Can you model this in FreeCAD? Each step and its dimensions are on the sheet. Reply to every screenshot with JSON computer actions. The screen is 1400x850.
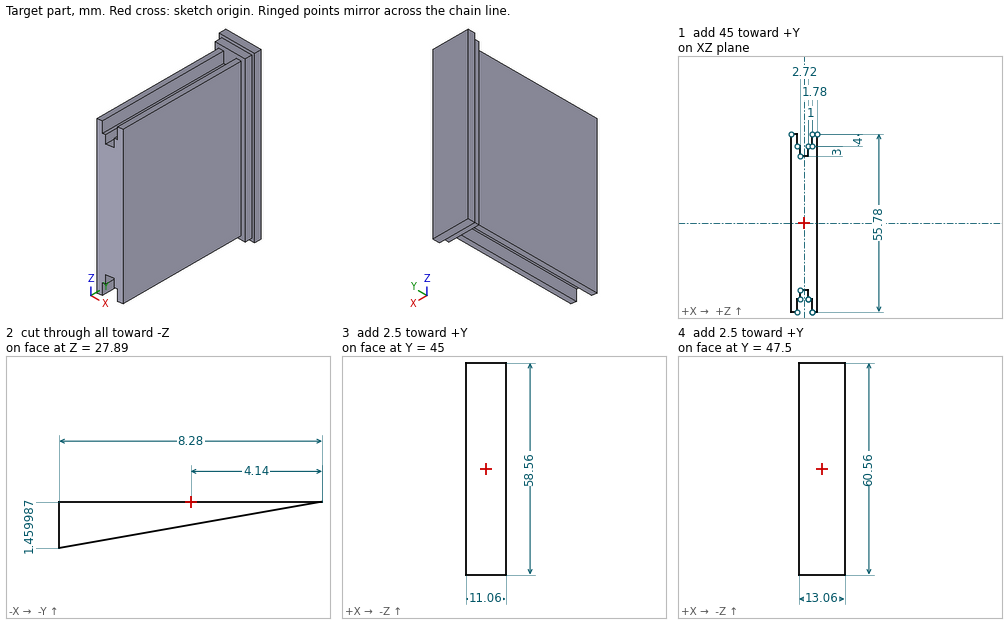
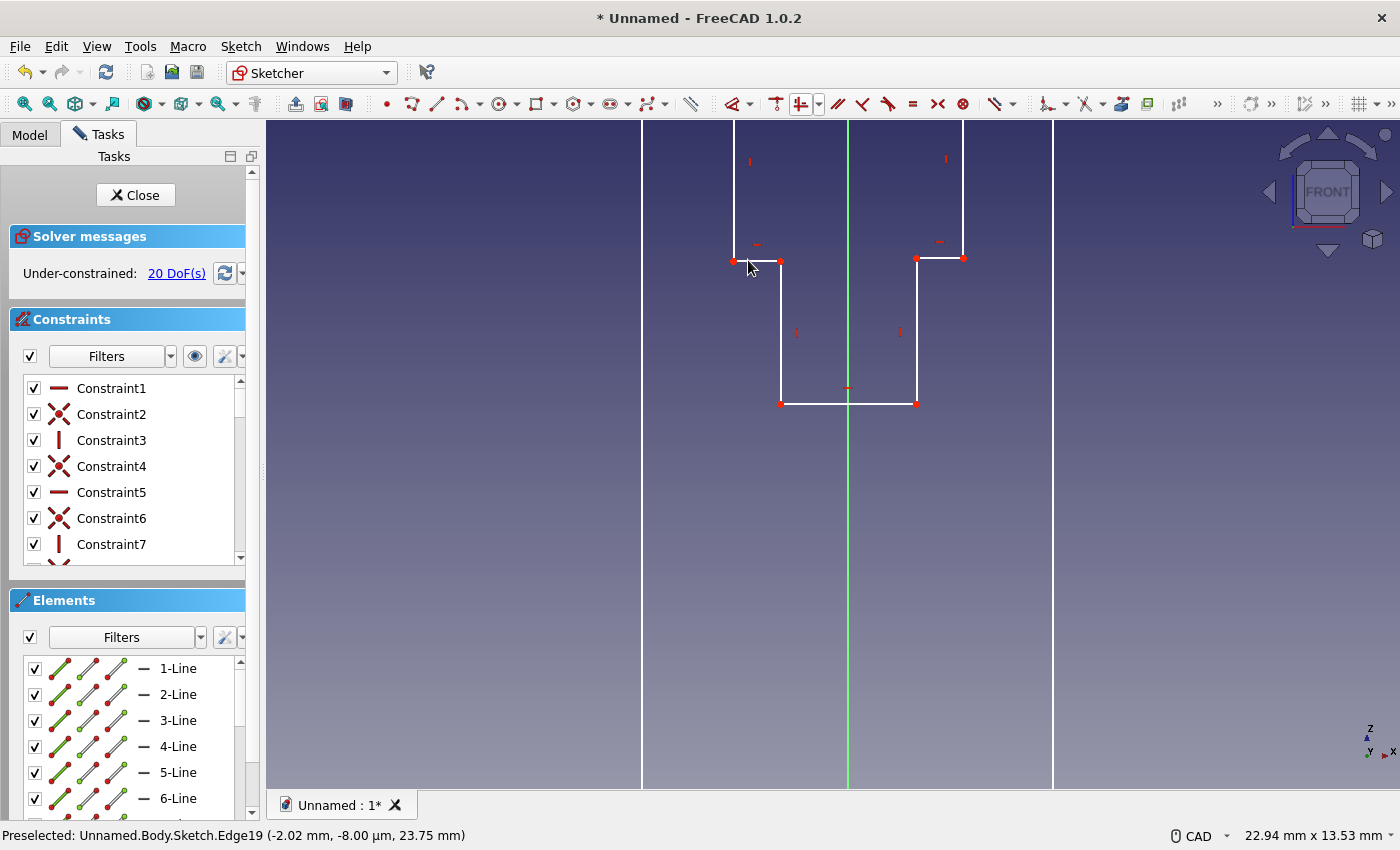
{"action": "scroll", "coordinate": [748, 260], "scroll_direction": "down", "scroll_amount": 9}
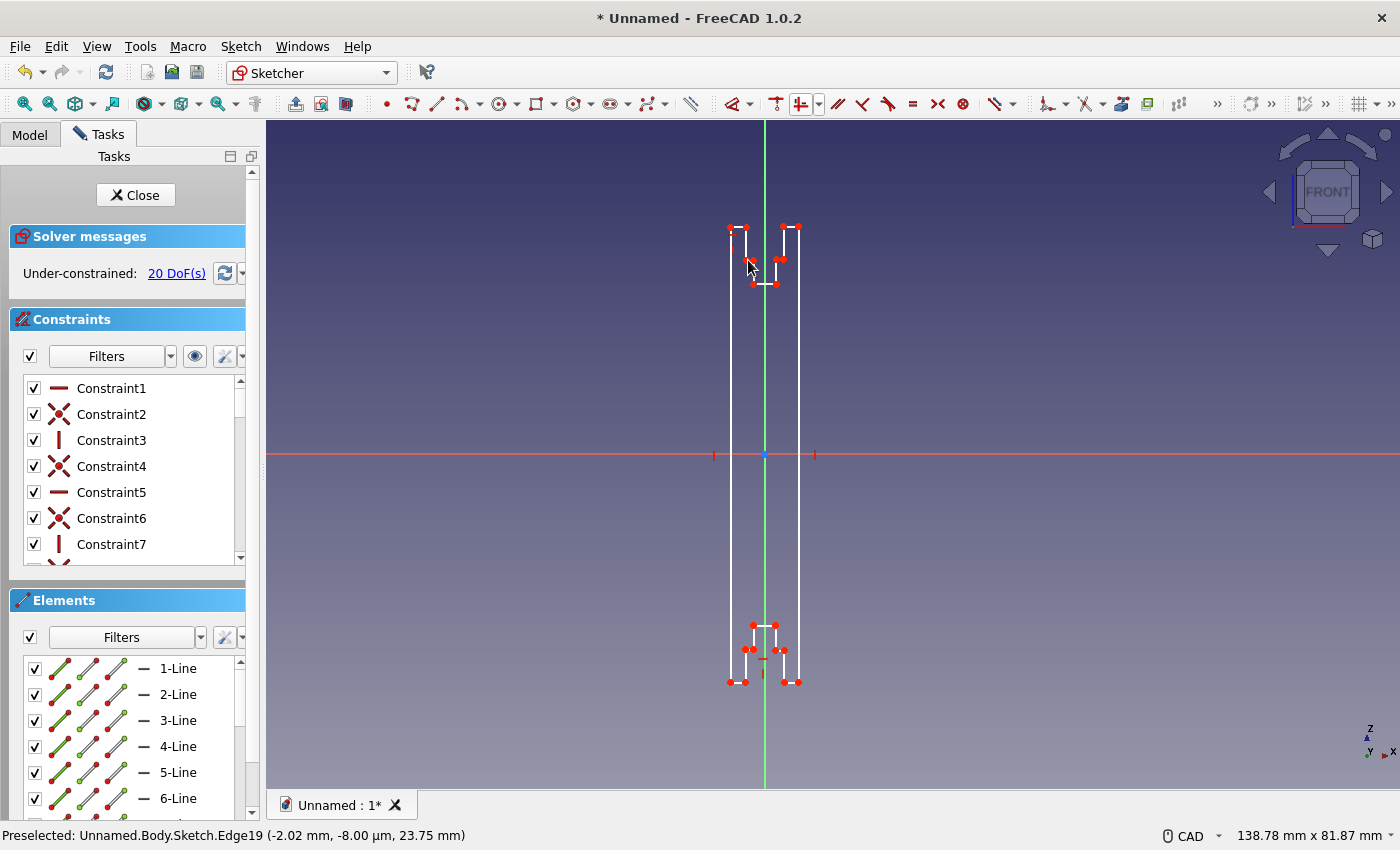
{"action": "left_click", "coordinate": [784, 227]}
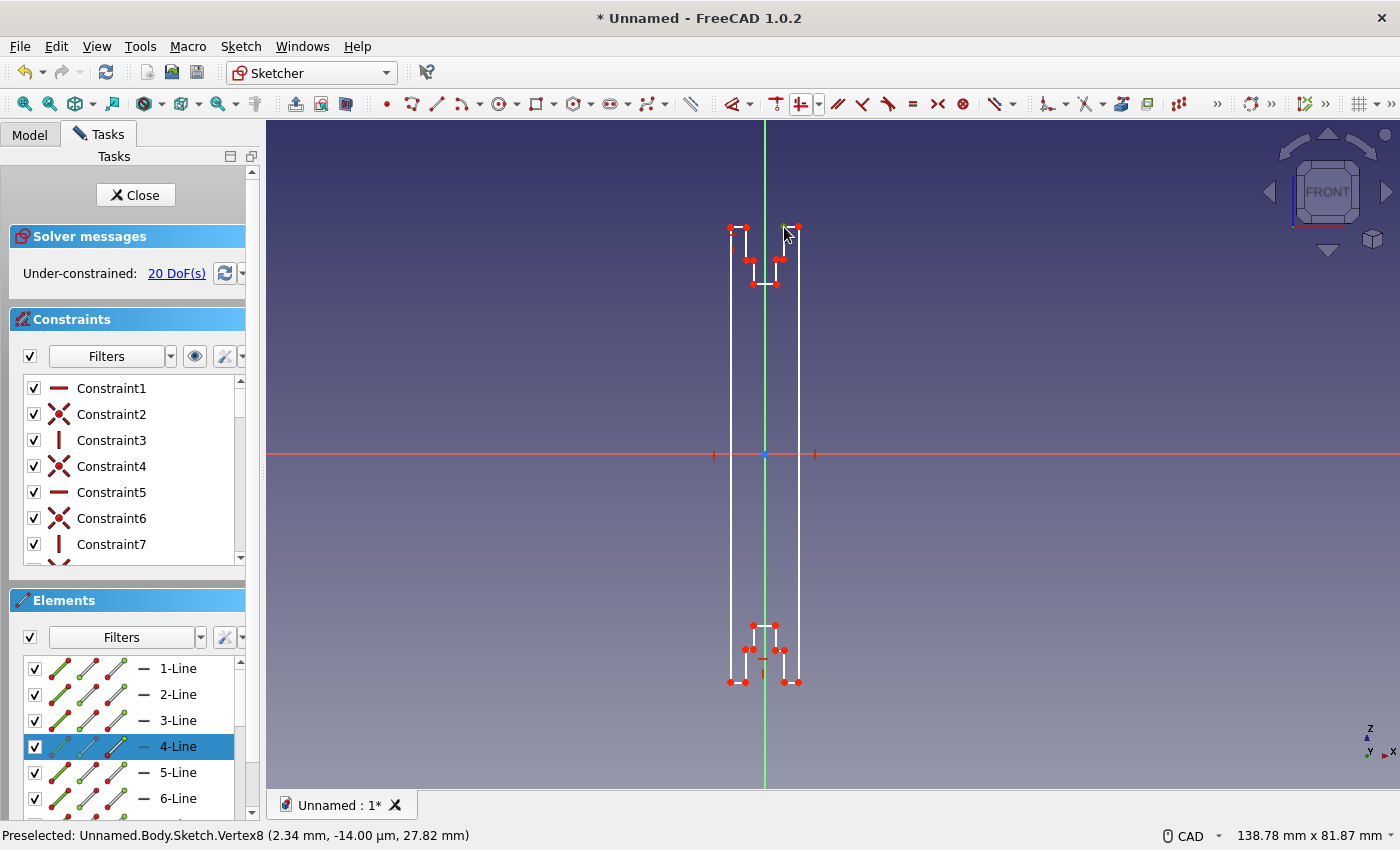
{"action": "left_click", "coordinate": [784, 683]}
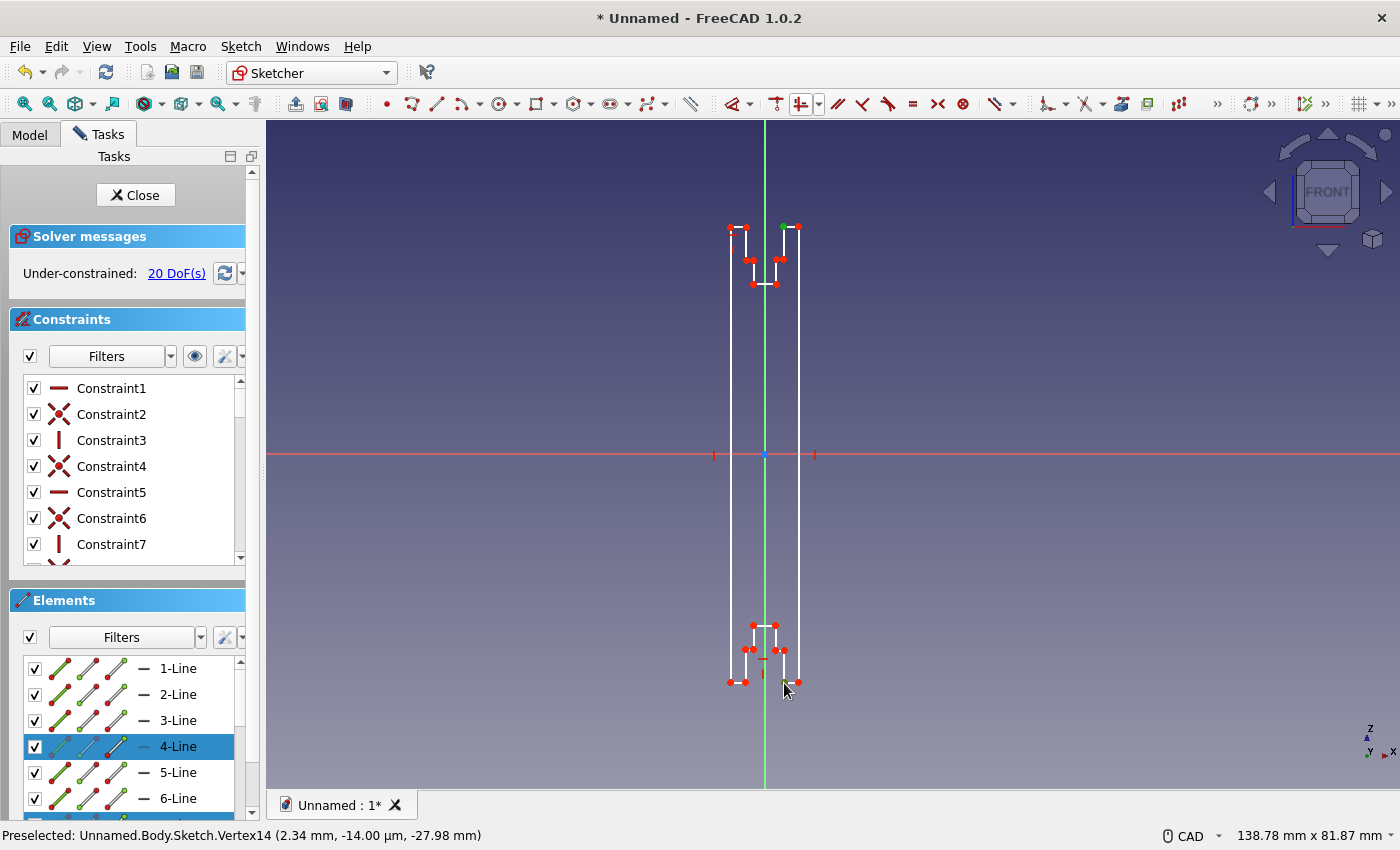
{"action": "left_click", "coordinate": [361, 454]}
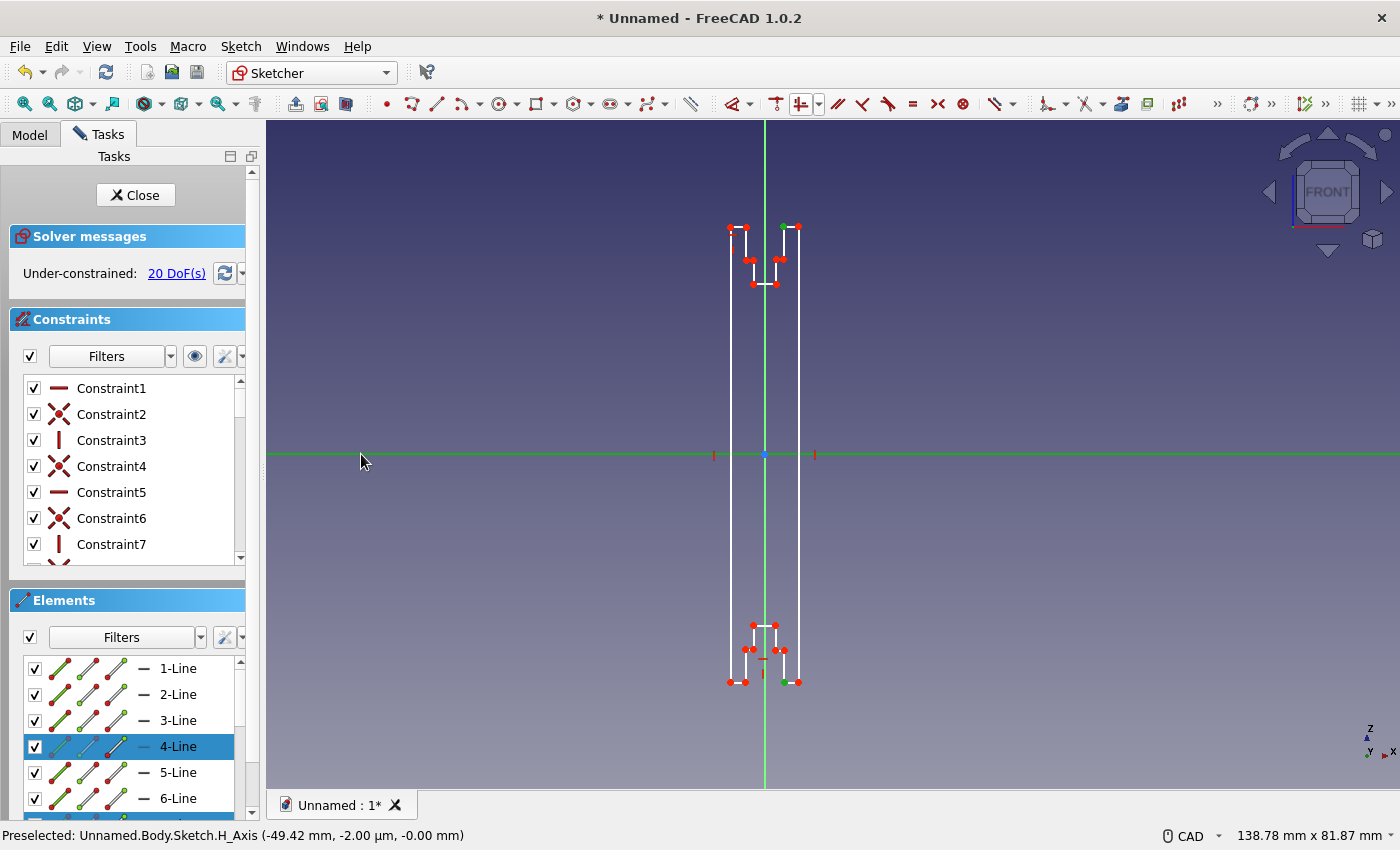
{"action": "left_click", "coordinate": [938, 104]}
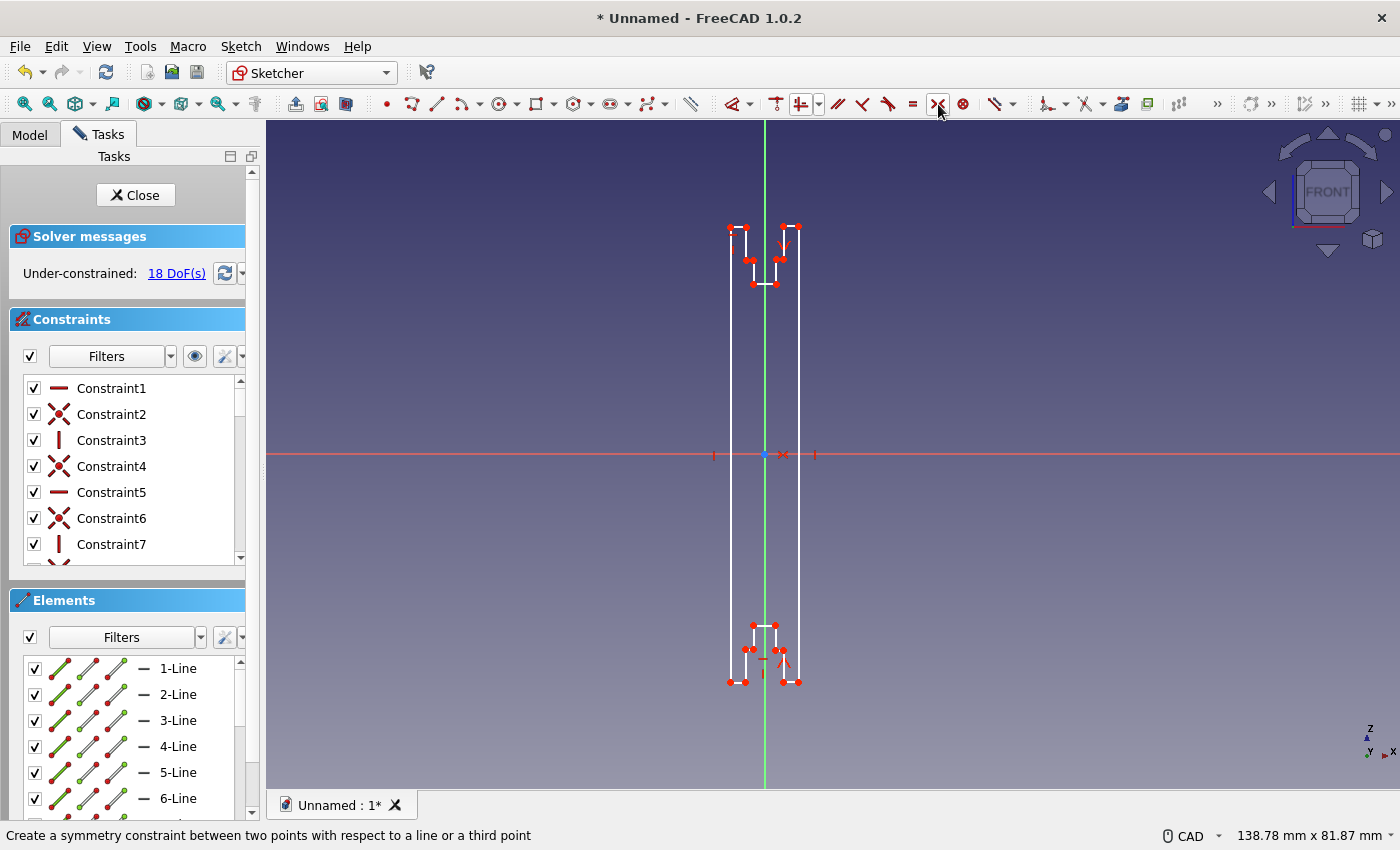
{"action": "scroll", "coordinate": [776, 260], "scroll_direction": "up", "scroll_amount": 3}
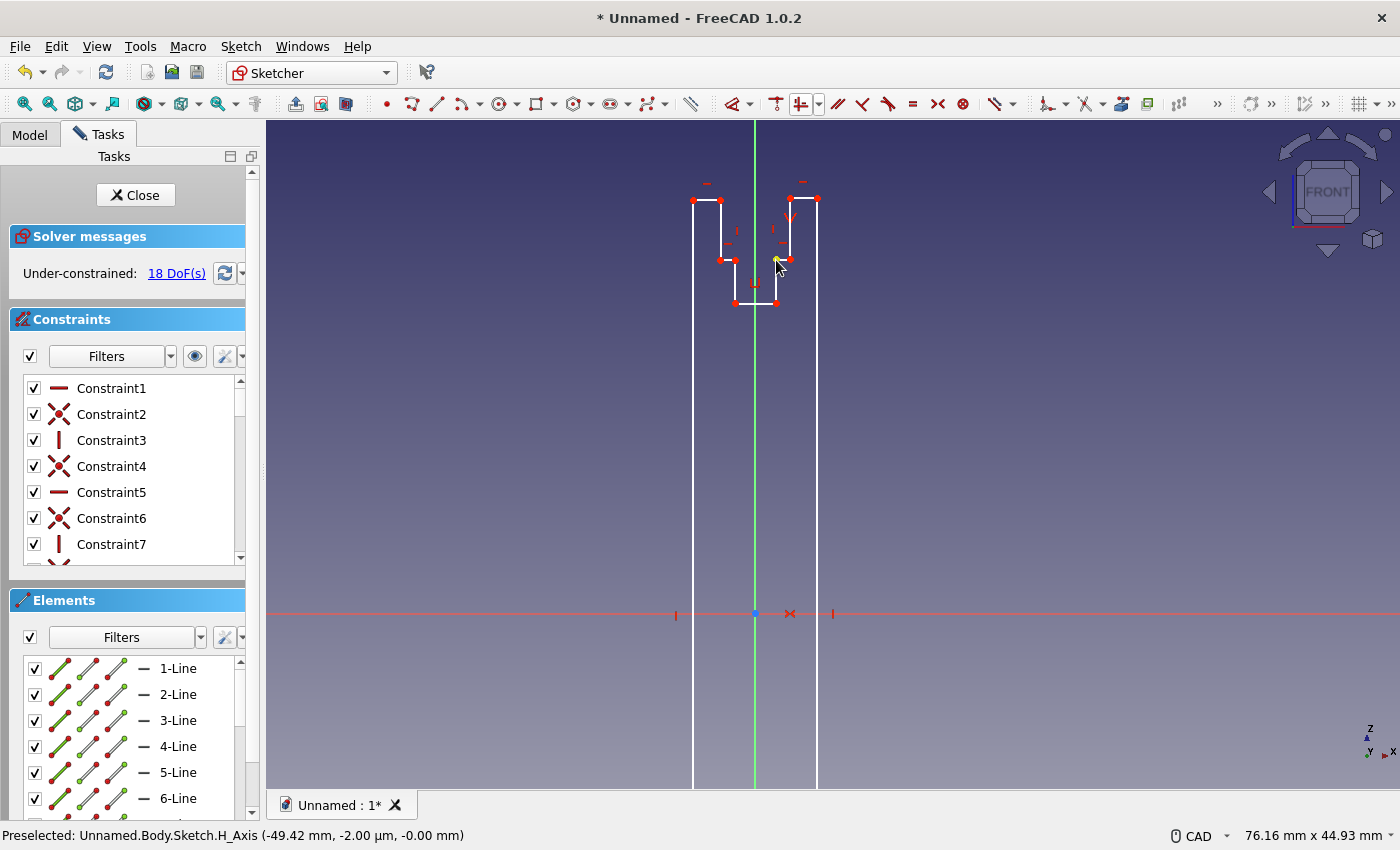
{"action": "left_click", "coordinate": [776, 260]}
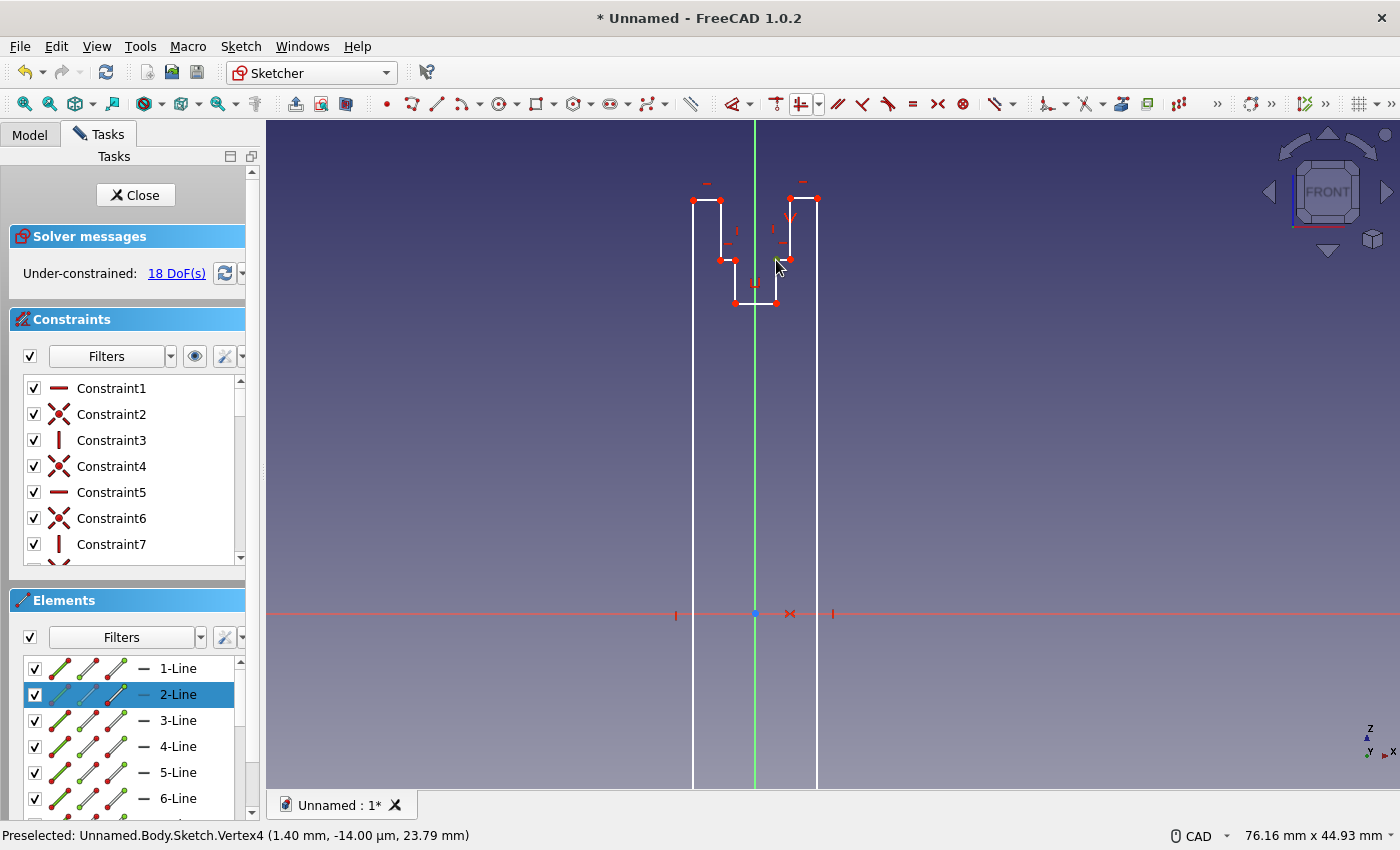
{"action": "scroll", "coordinate": [776, 261], "scroll_direction": "down", "scroll_amount": 3}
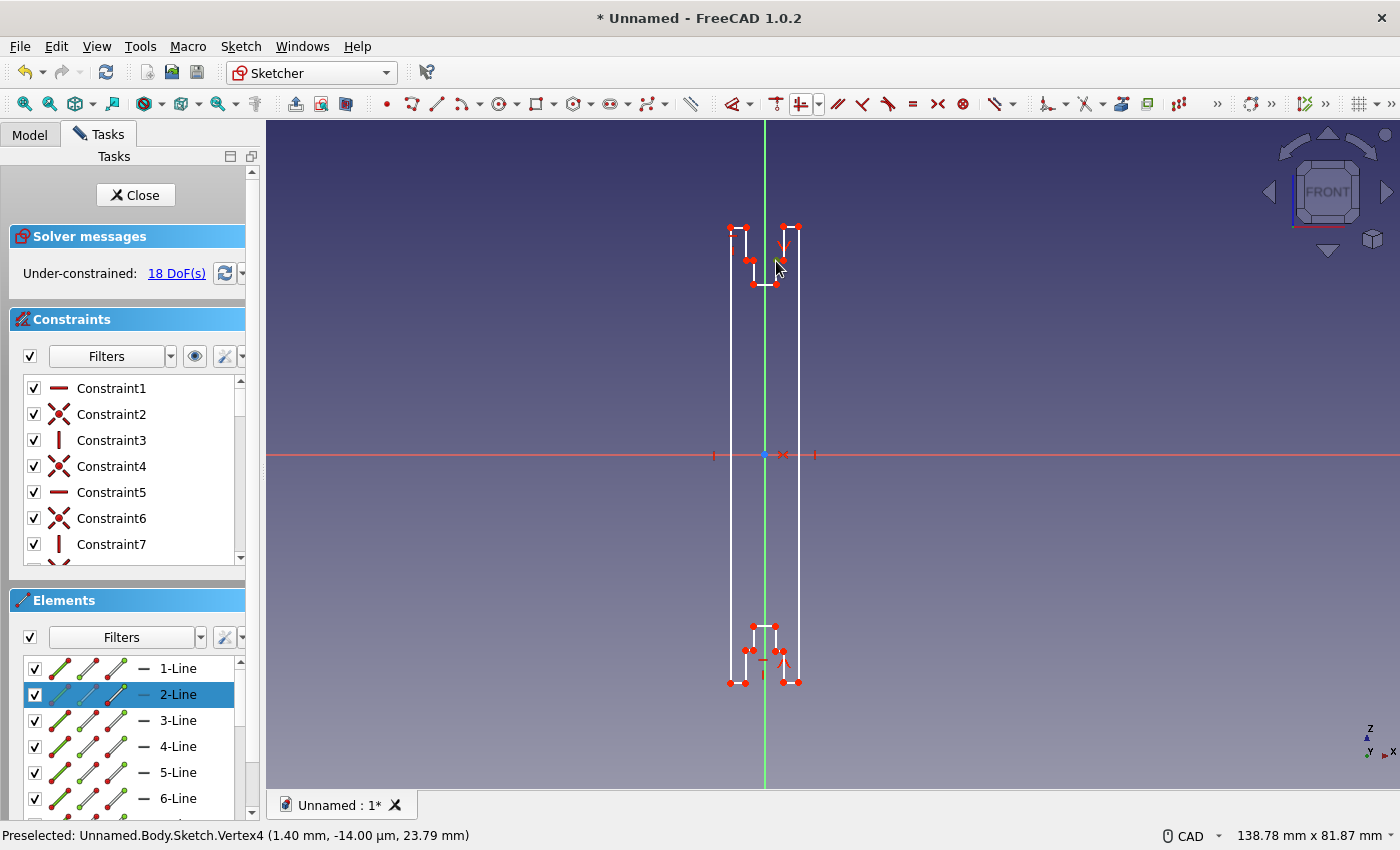
{"action": "scroll", "coordinate": [776, 651], "scroll_direction": "up", "scroll_amount": 3}